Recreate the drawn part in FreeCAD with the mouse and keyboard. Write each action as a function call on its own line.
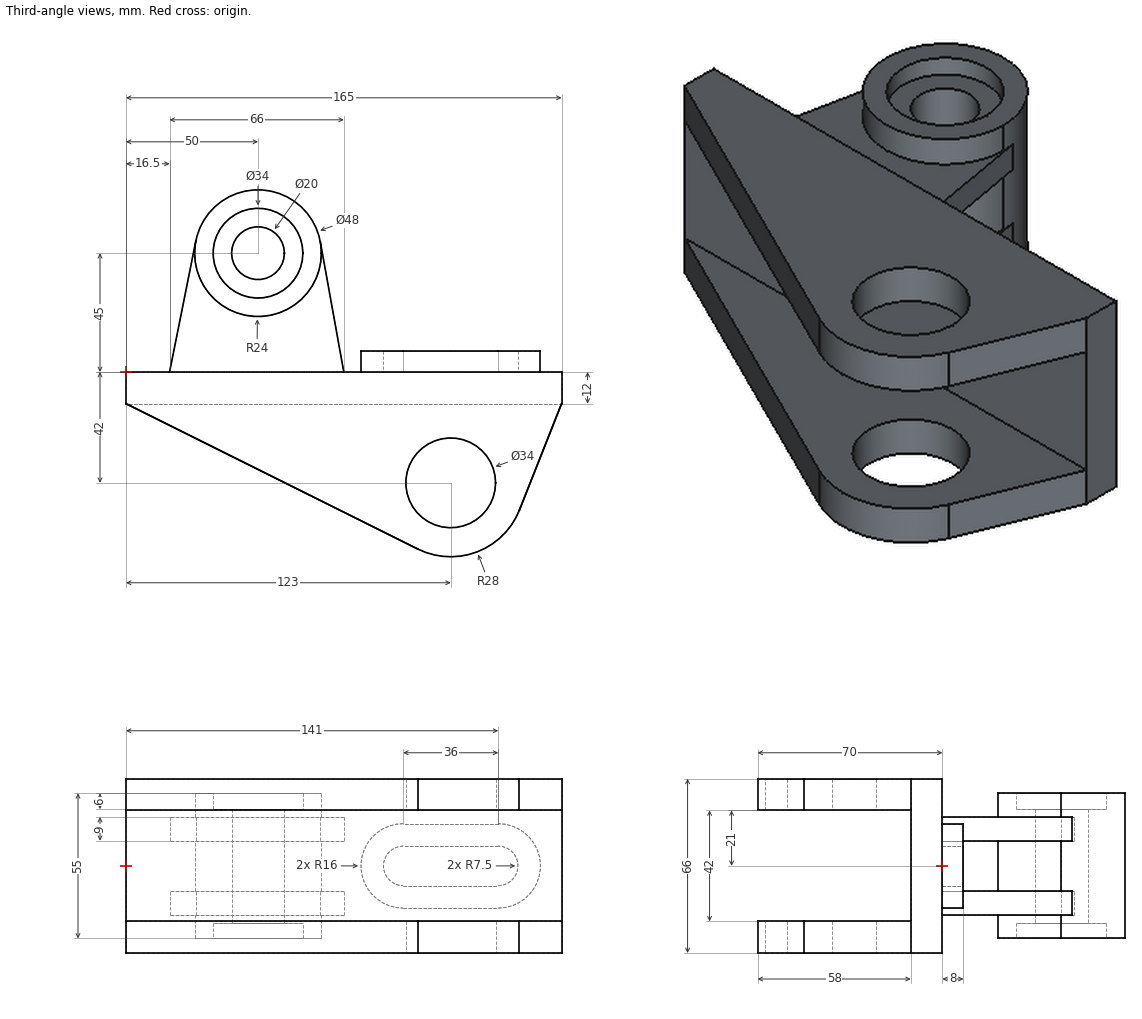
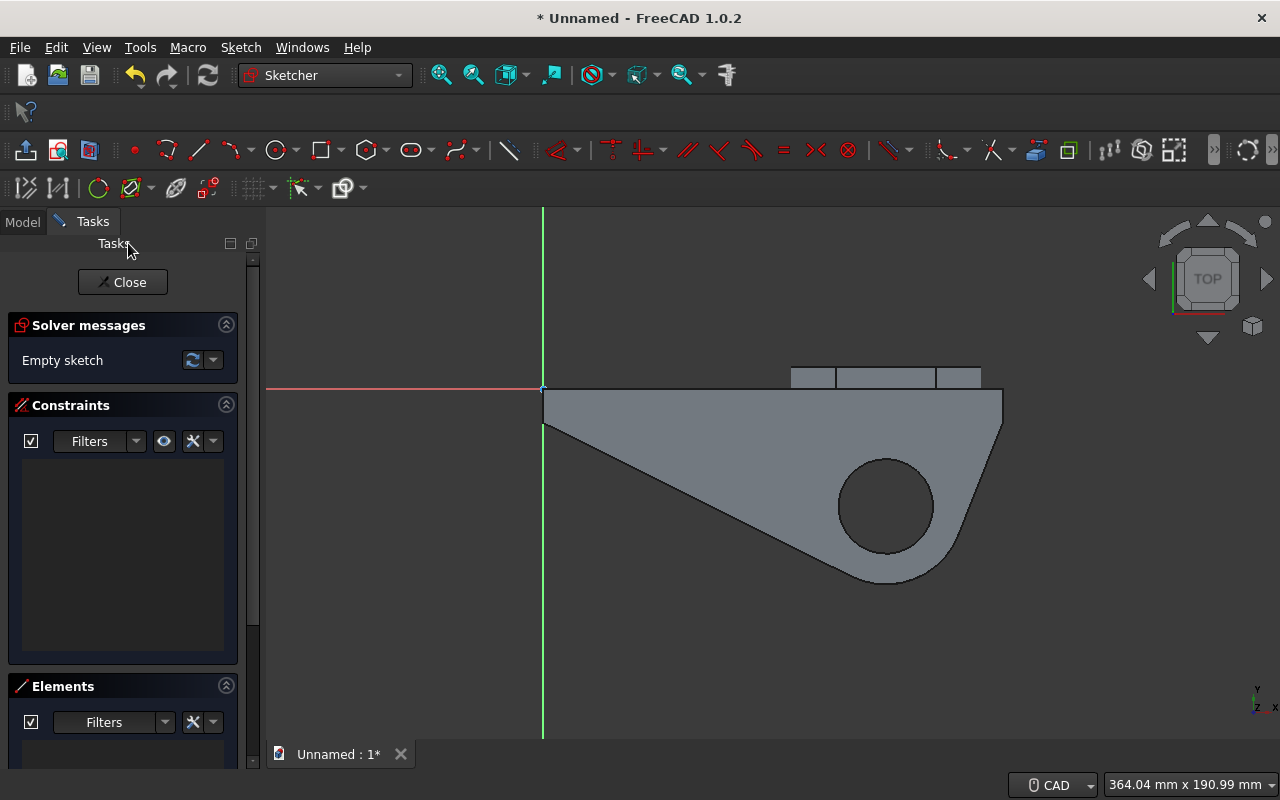
scroll(704, 473, down, 5)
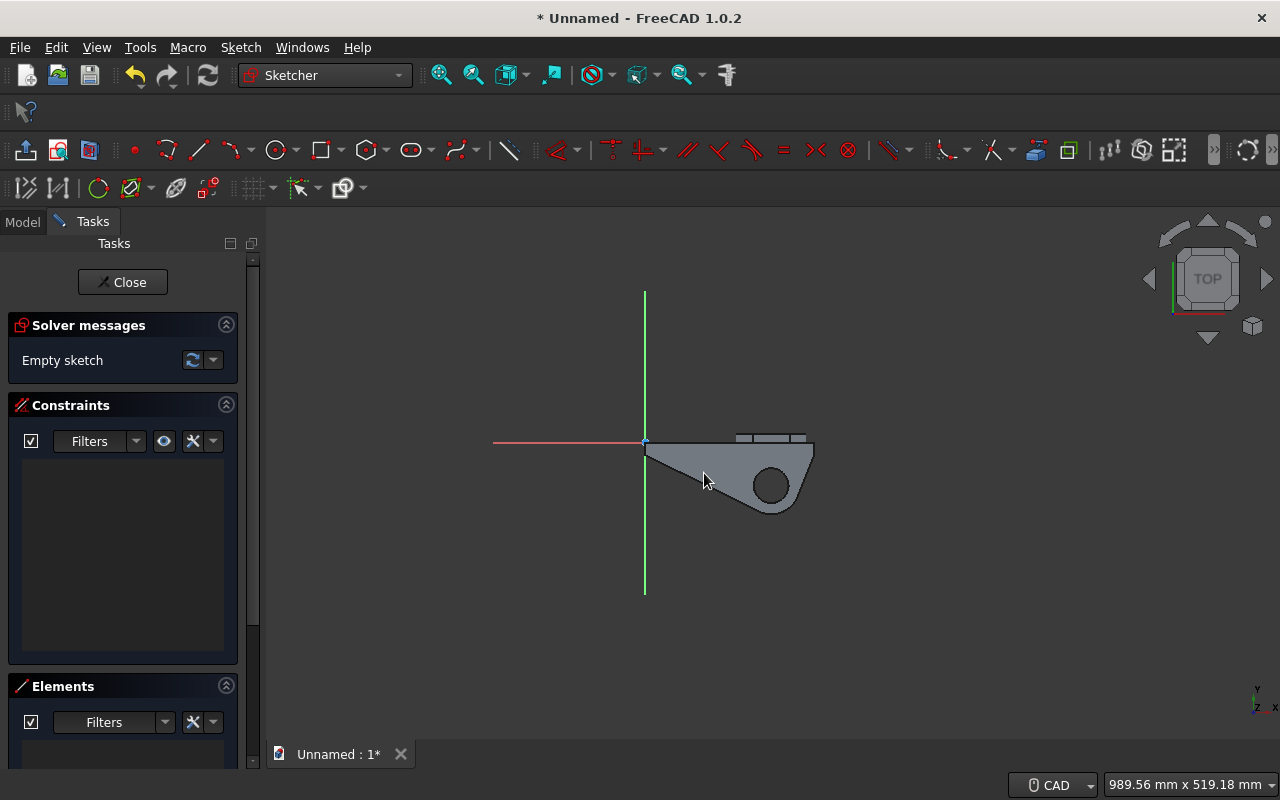
scroll(678, 391, up, 8)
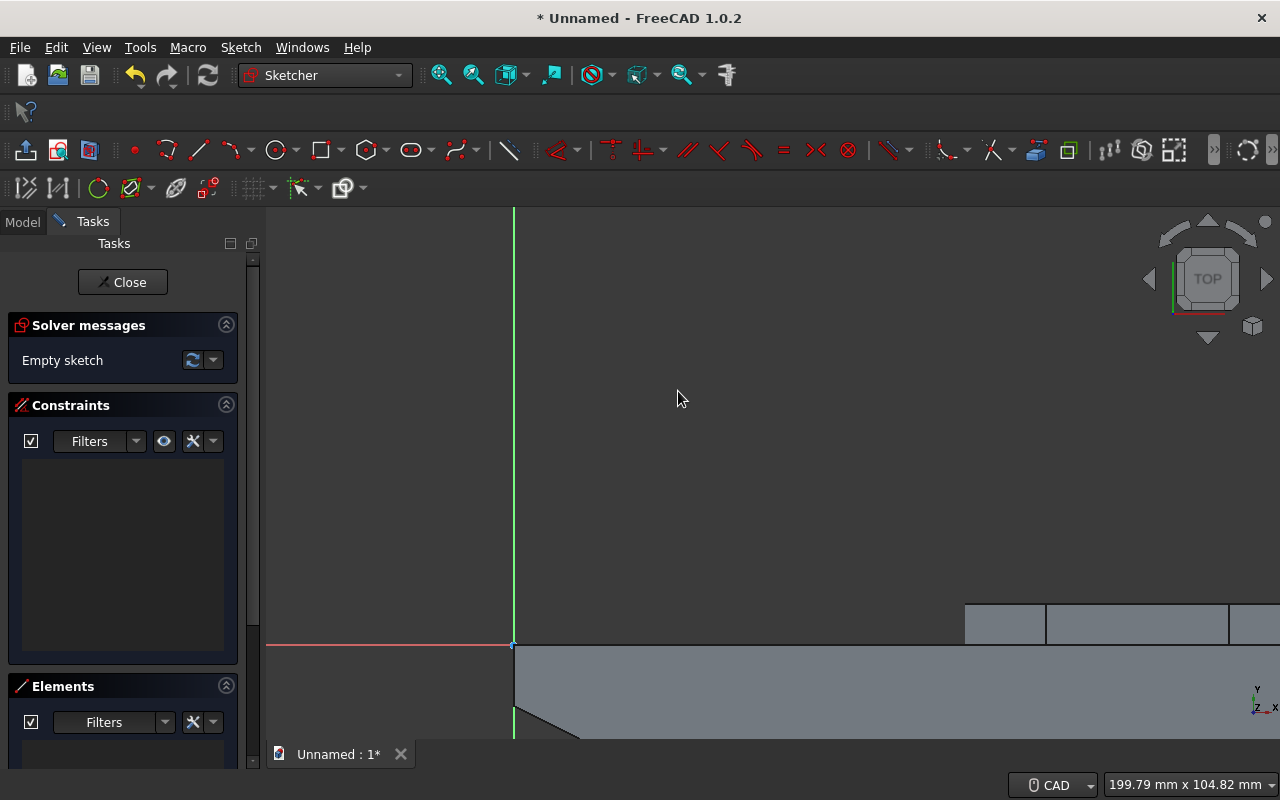
key(g)
key(c)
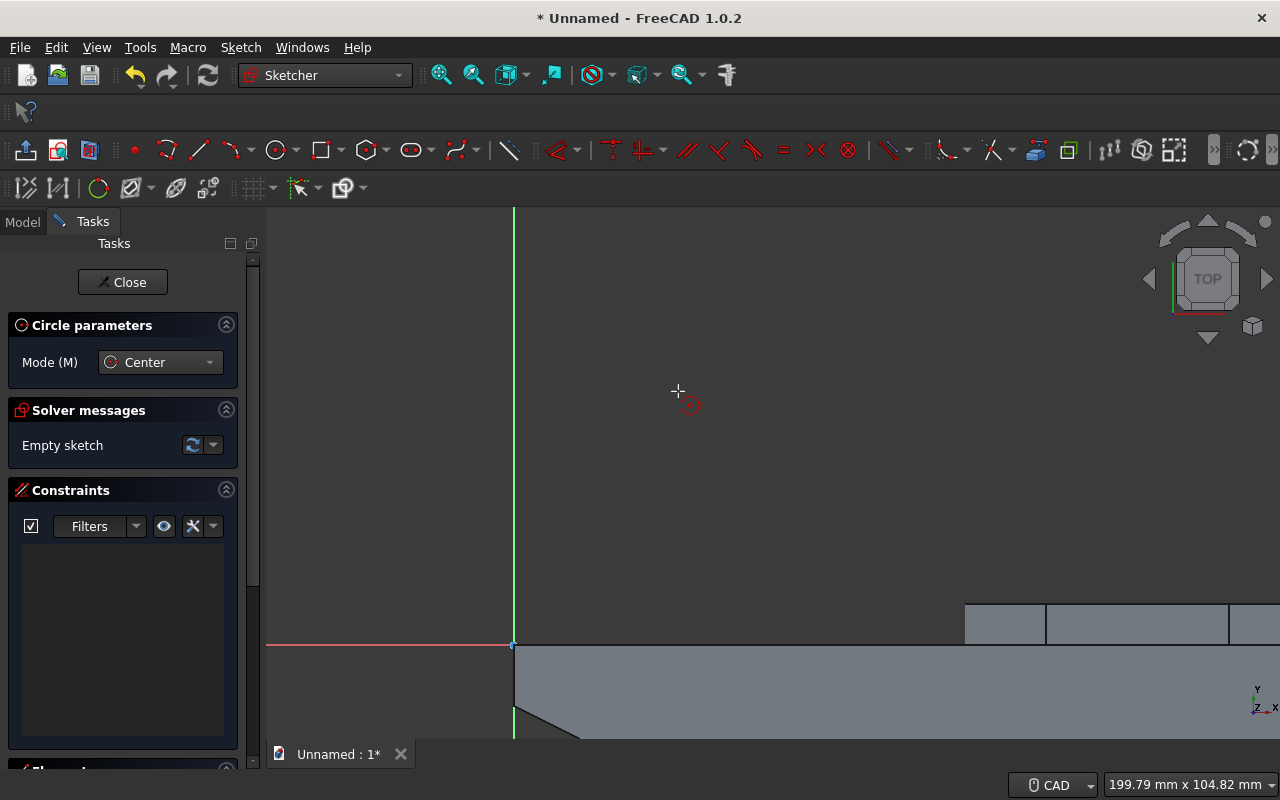
click(767, 417)
move(853, 331)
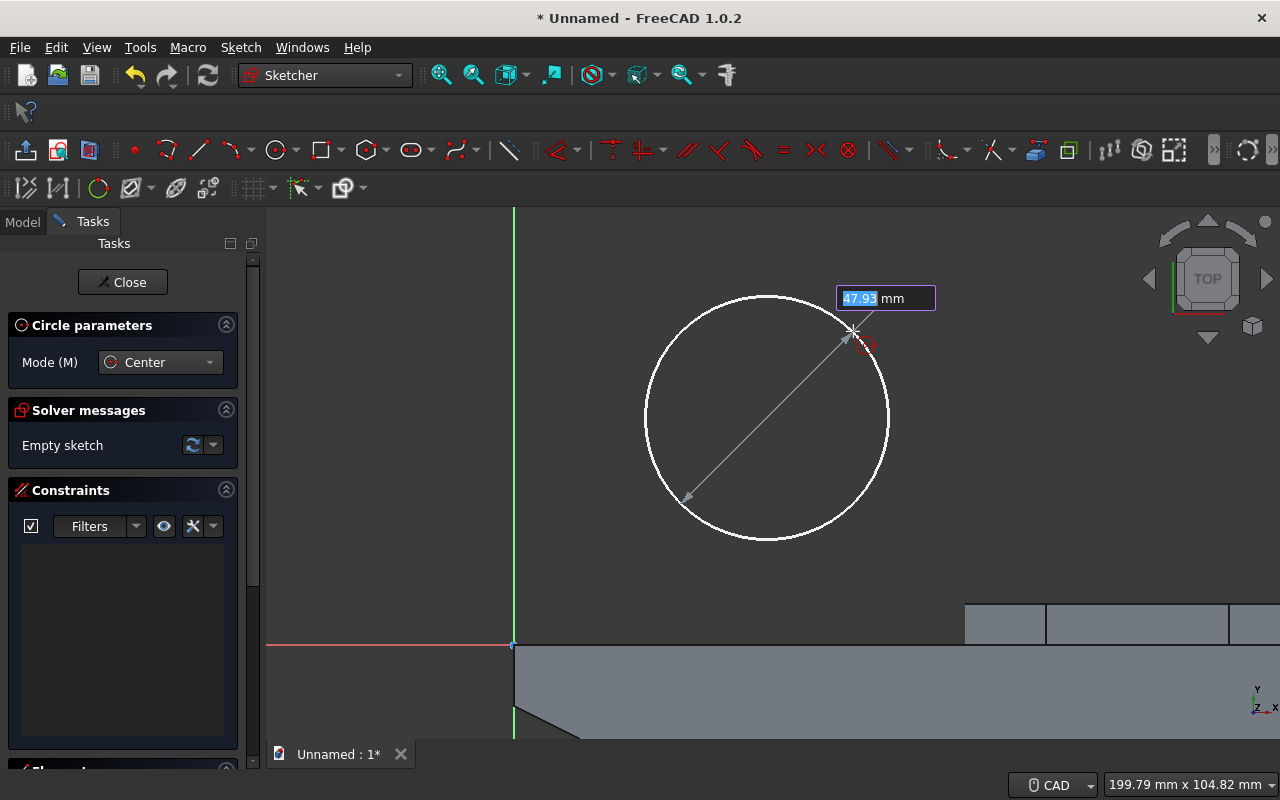
text(48)
key(Return)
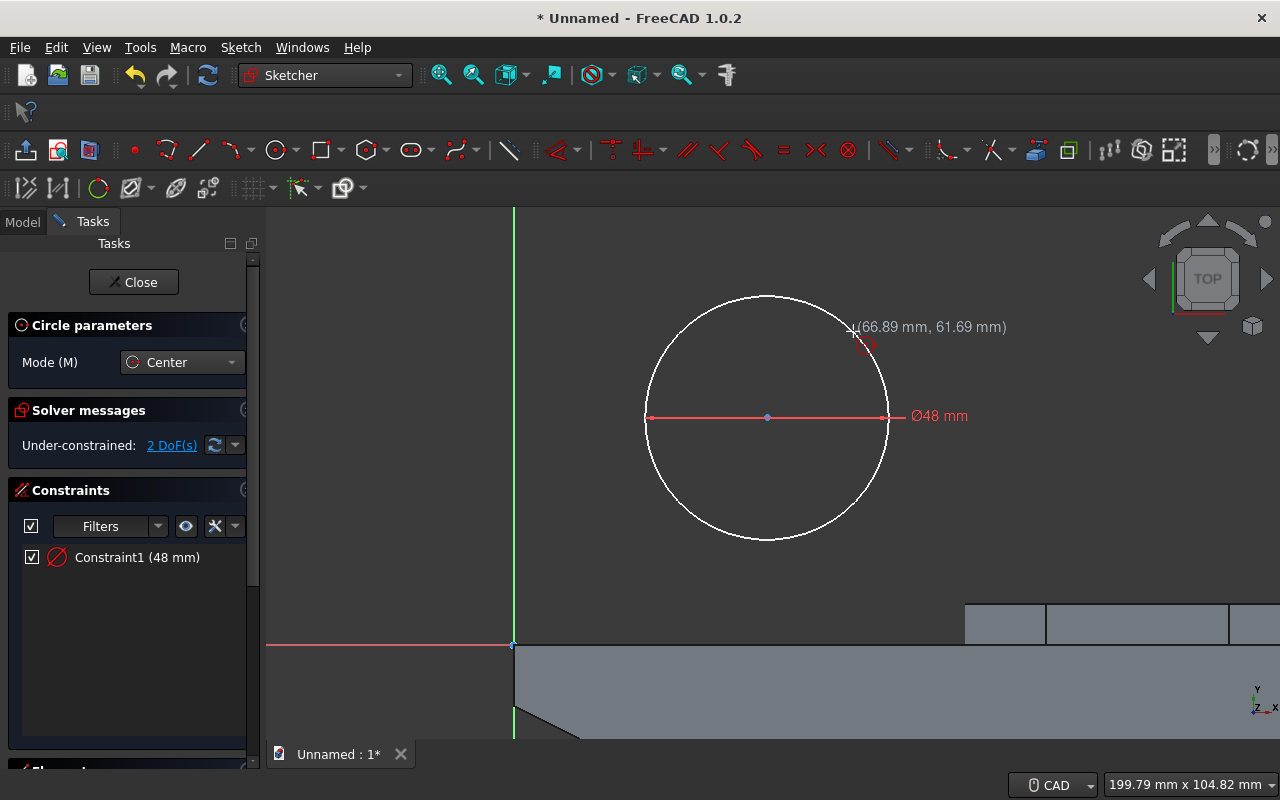
click(767, 418)
move(803, 381)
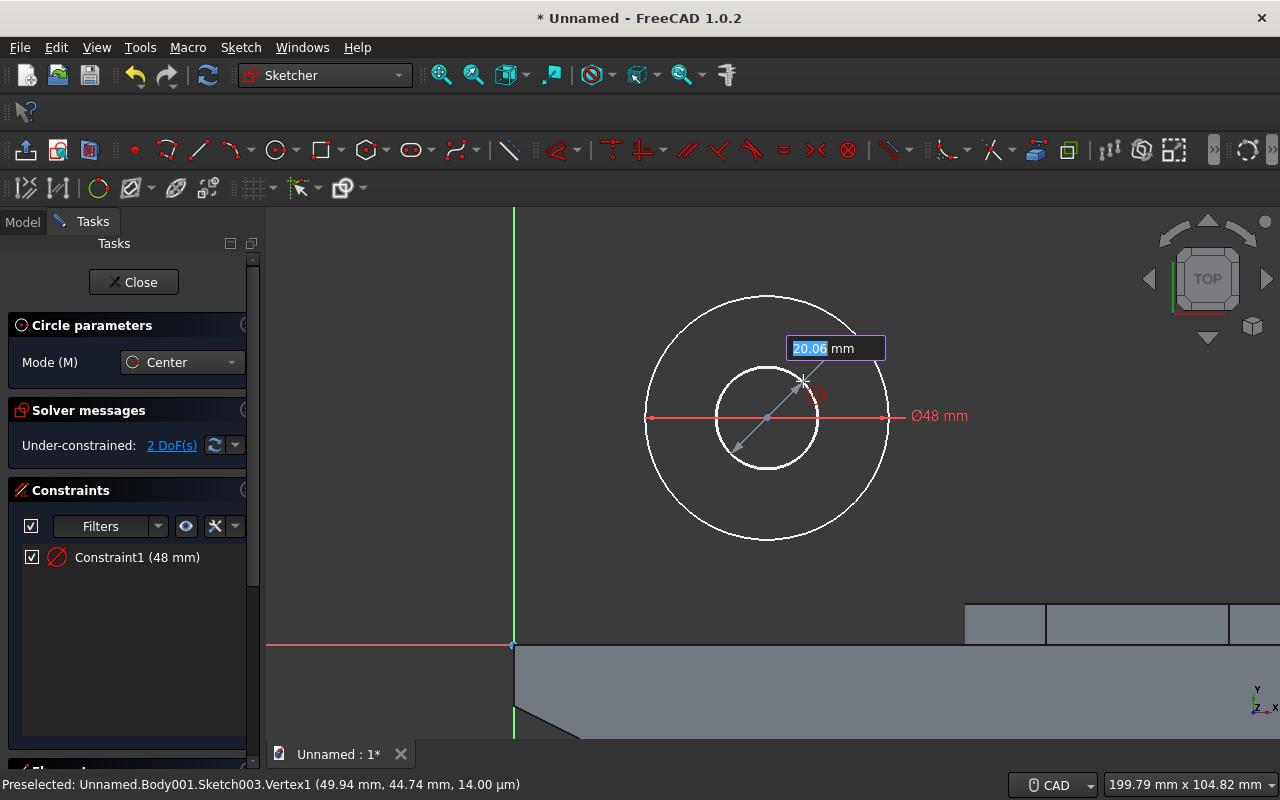
text(20)
key(Return)
key(Escape)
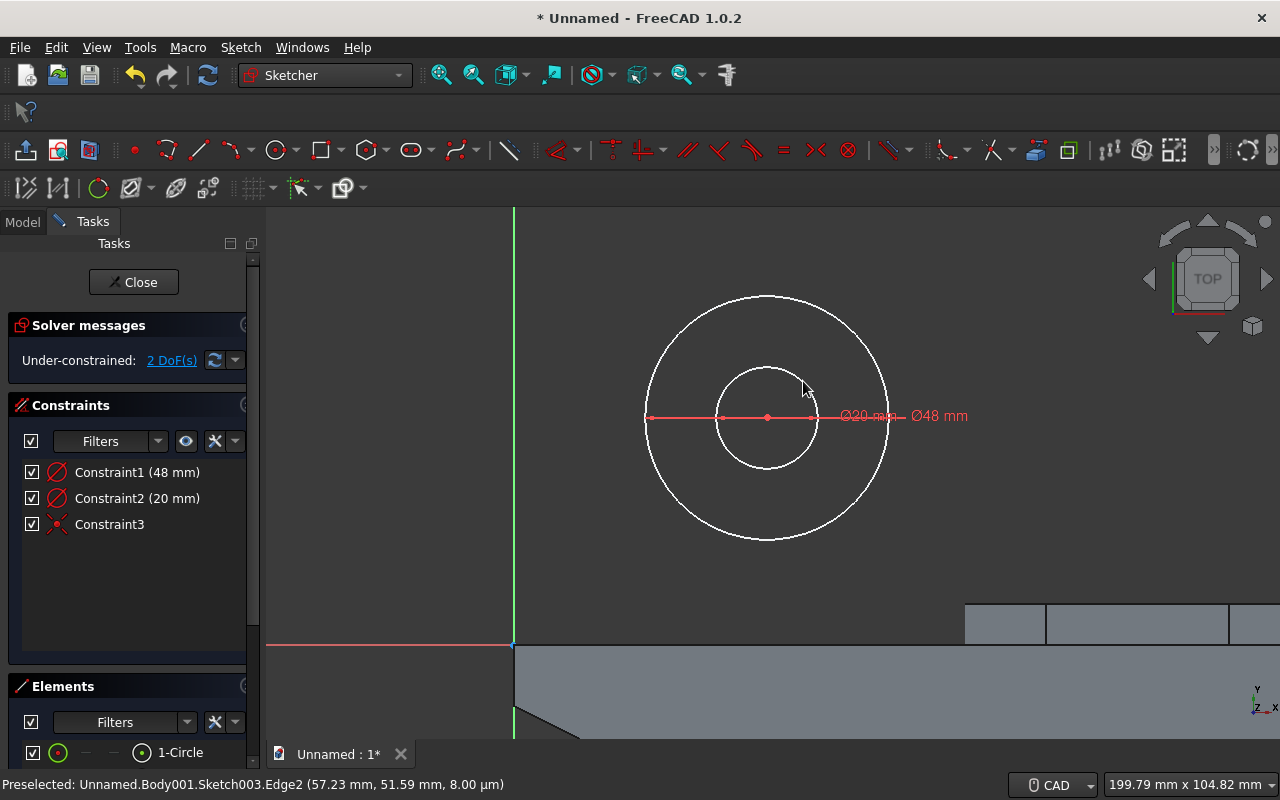
key(d)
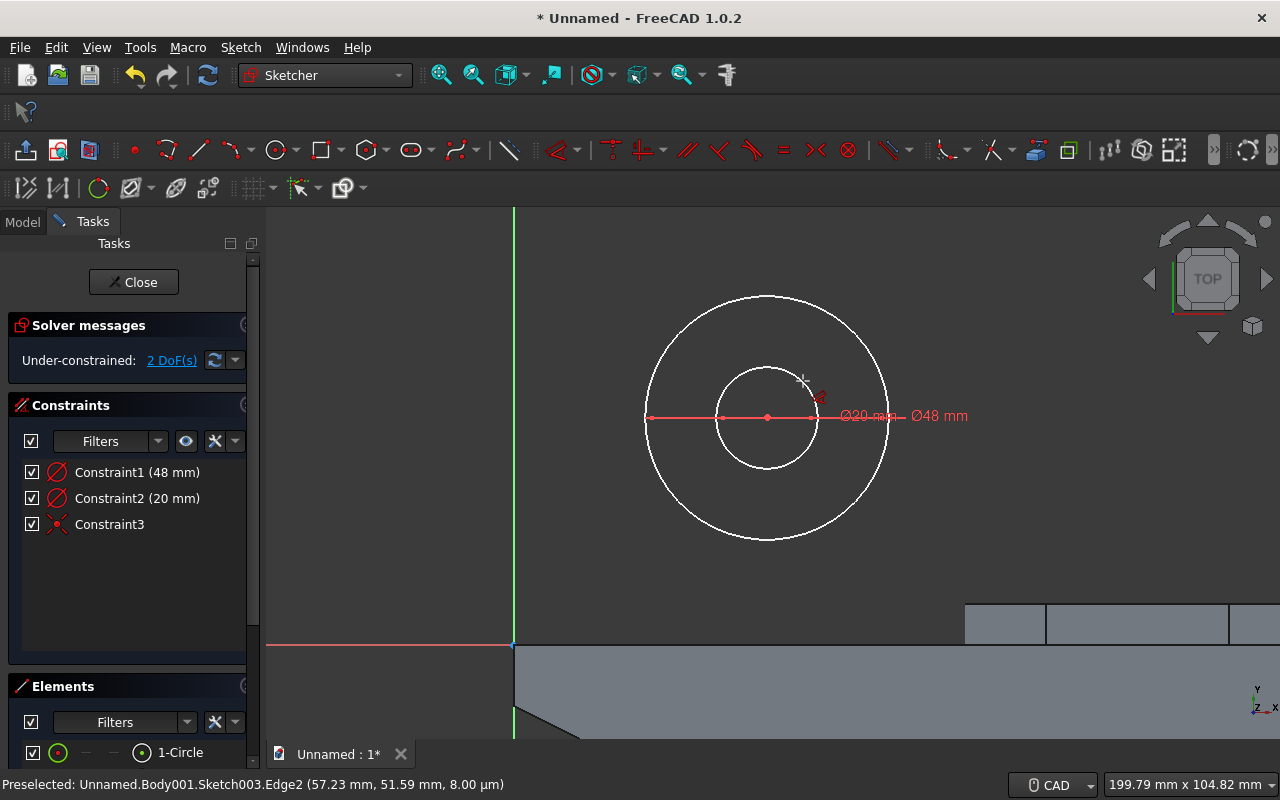
click(767, 418)
click(640, 679)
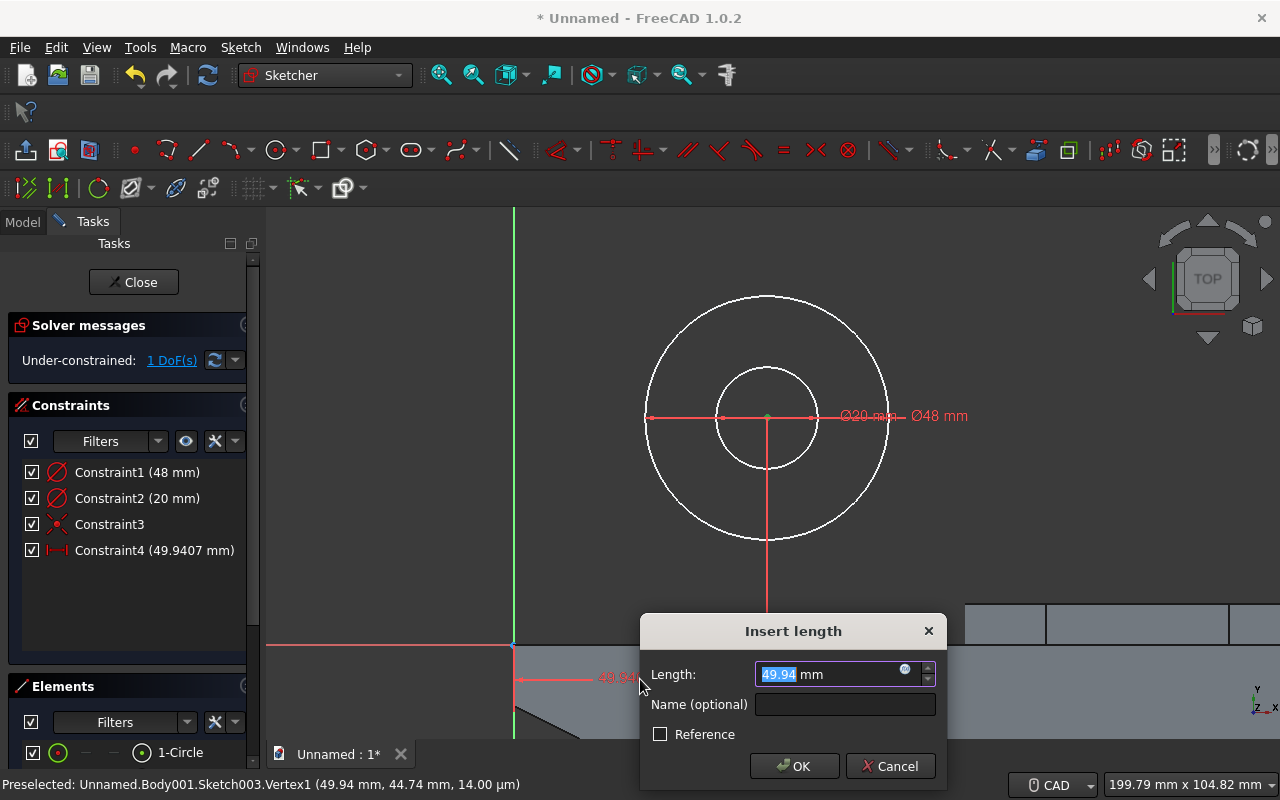
text(50)
key(Return)